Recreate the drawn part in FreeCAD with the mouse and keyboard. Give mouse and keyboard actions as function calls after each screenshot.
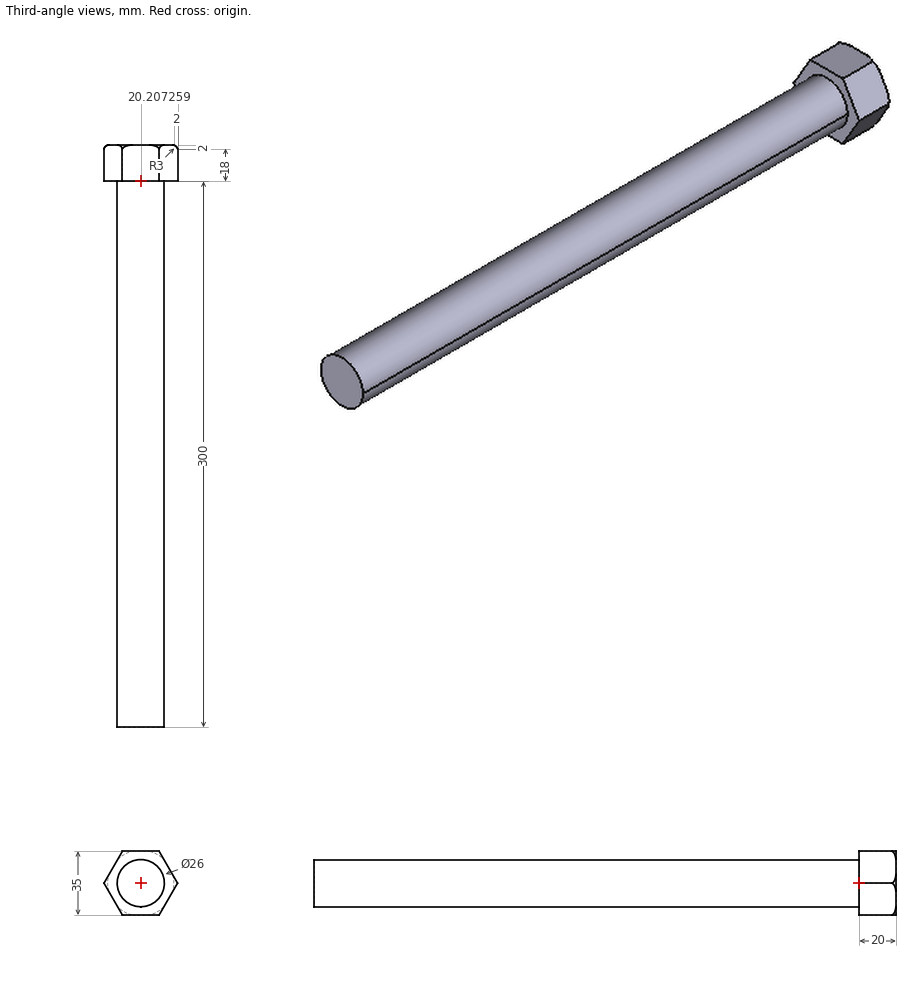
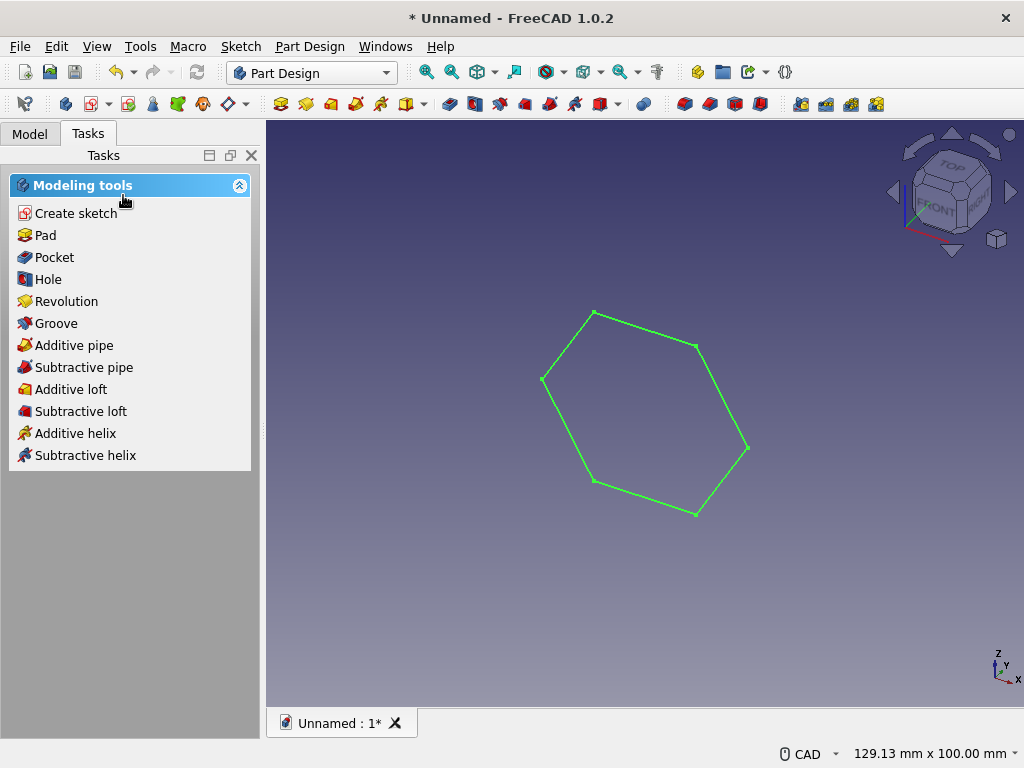
click(281, 104)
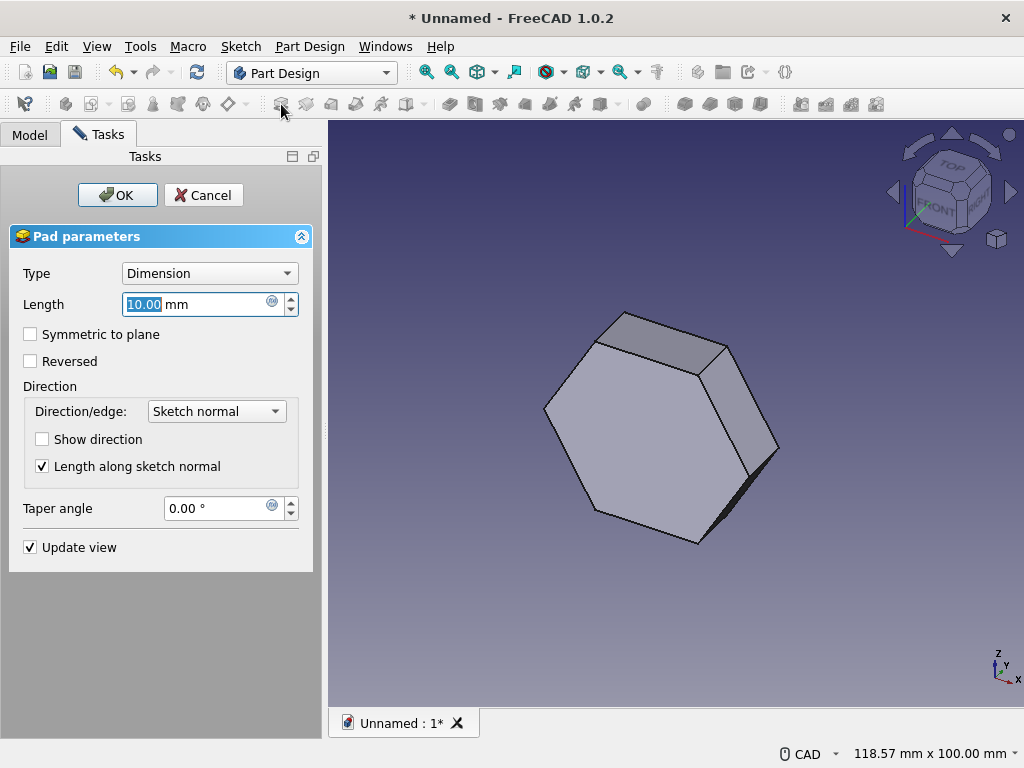
text(20)
key(Tab)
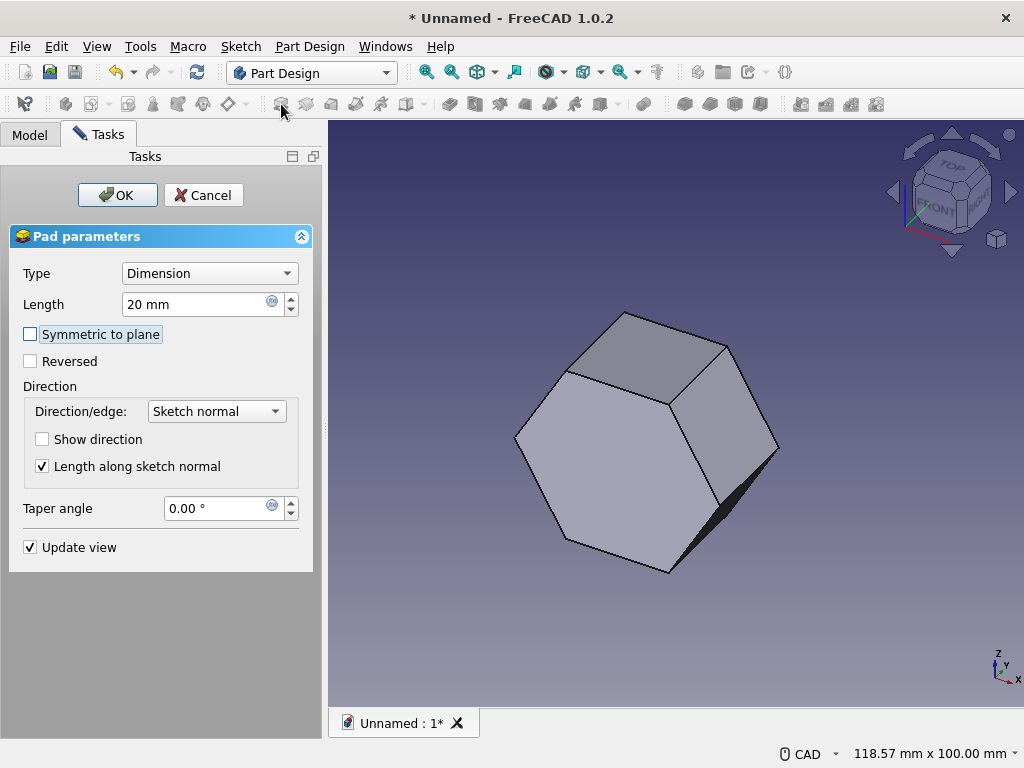
click(31, 361)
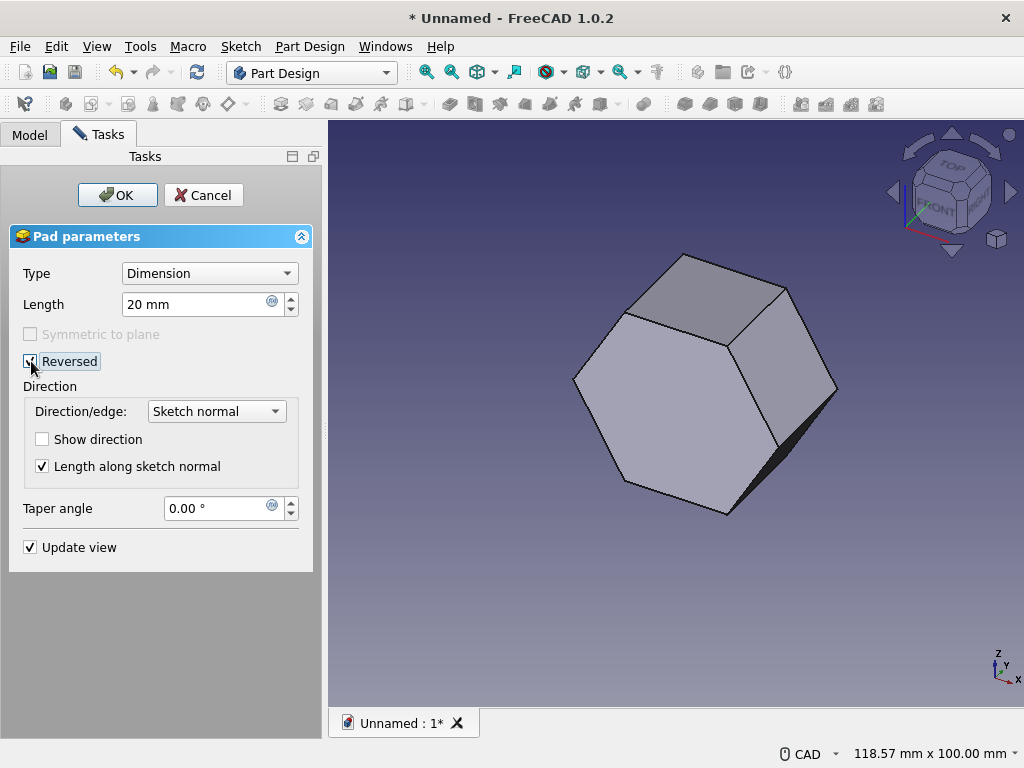
click(118, 195)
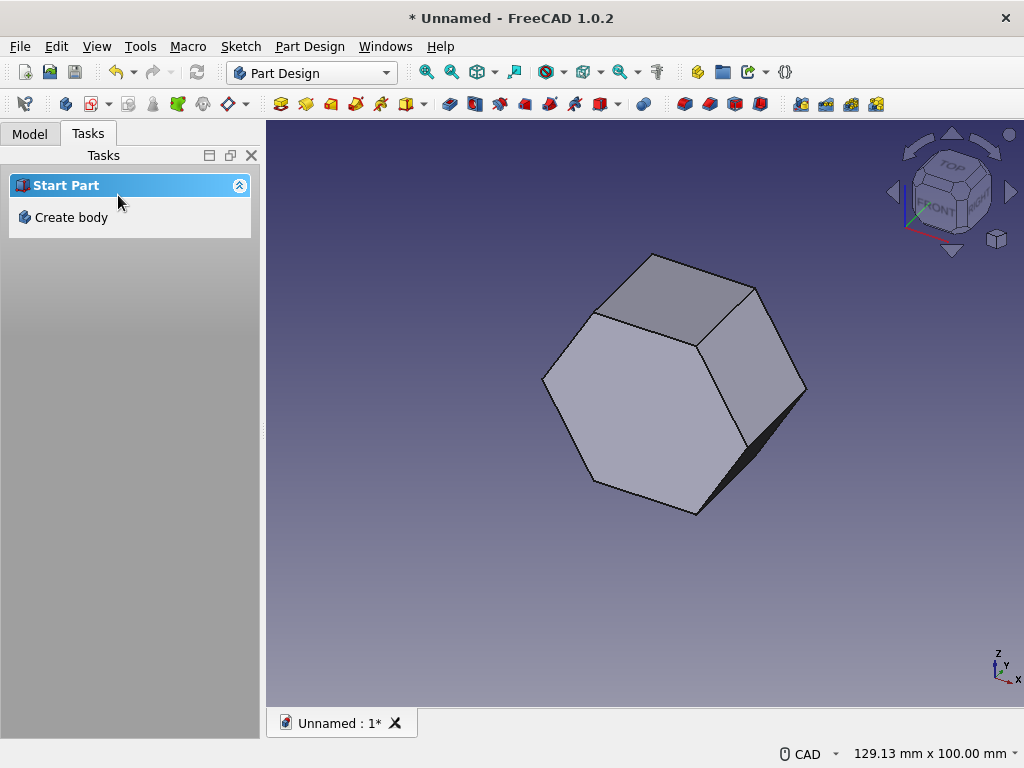
click(90, 104)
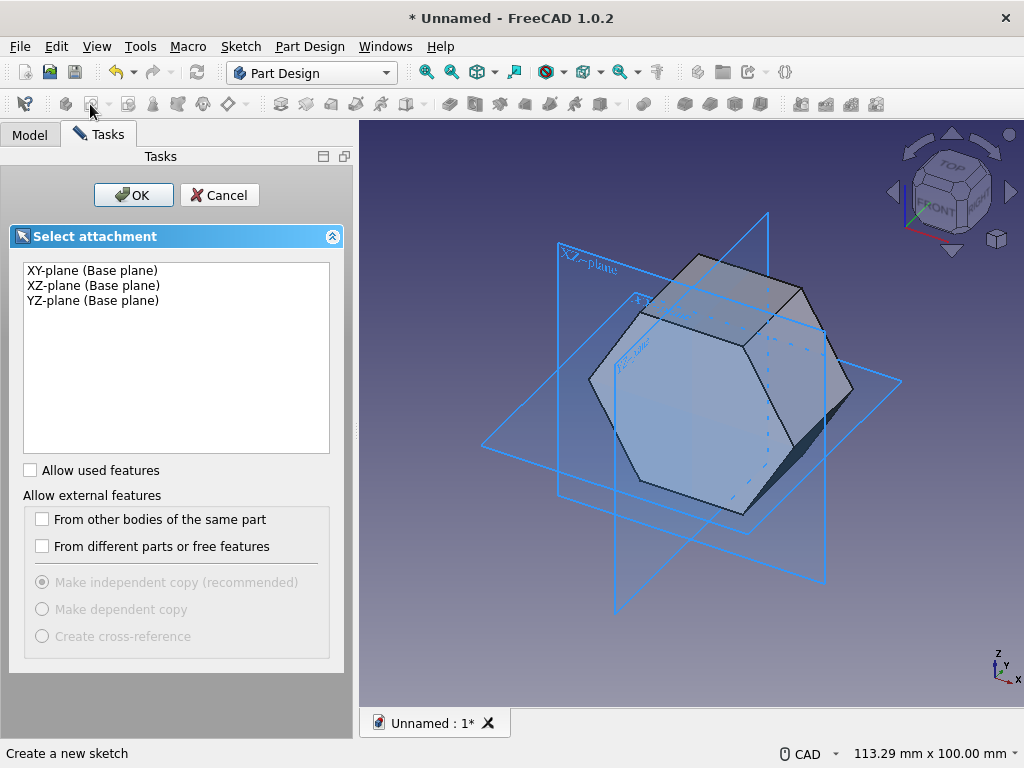
click(84, 286)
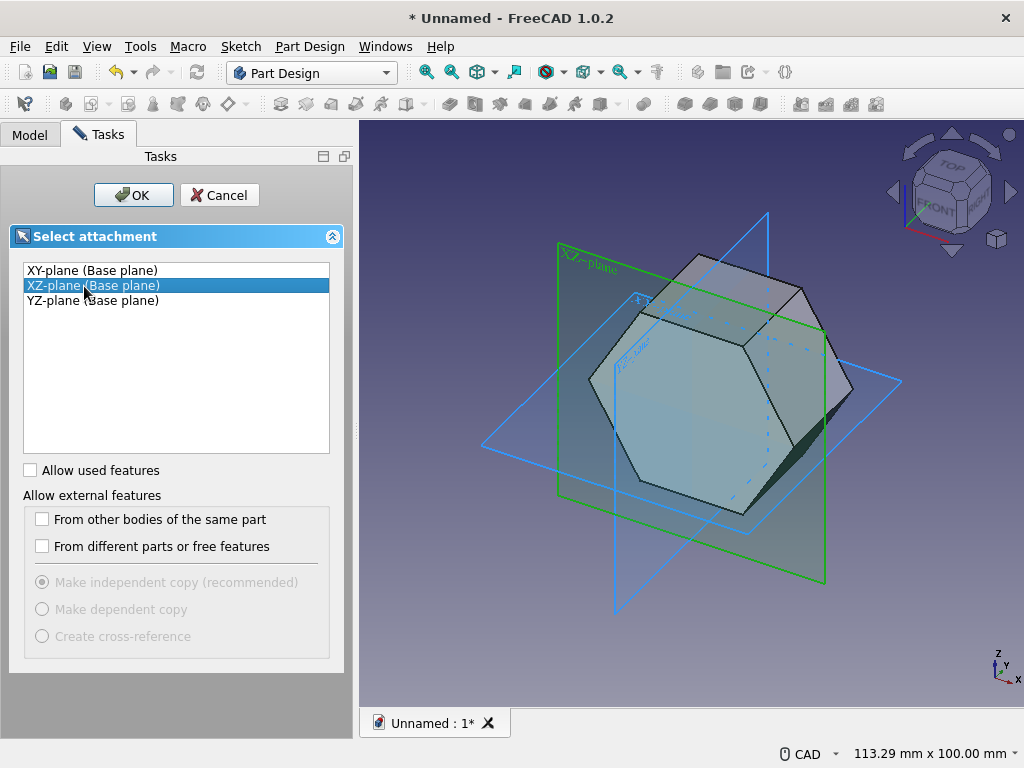
click(134, 195)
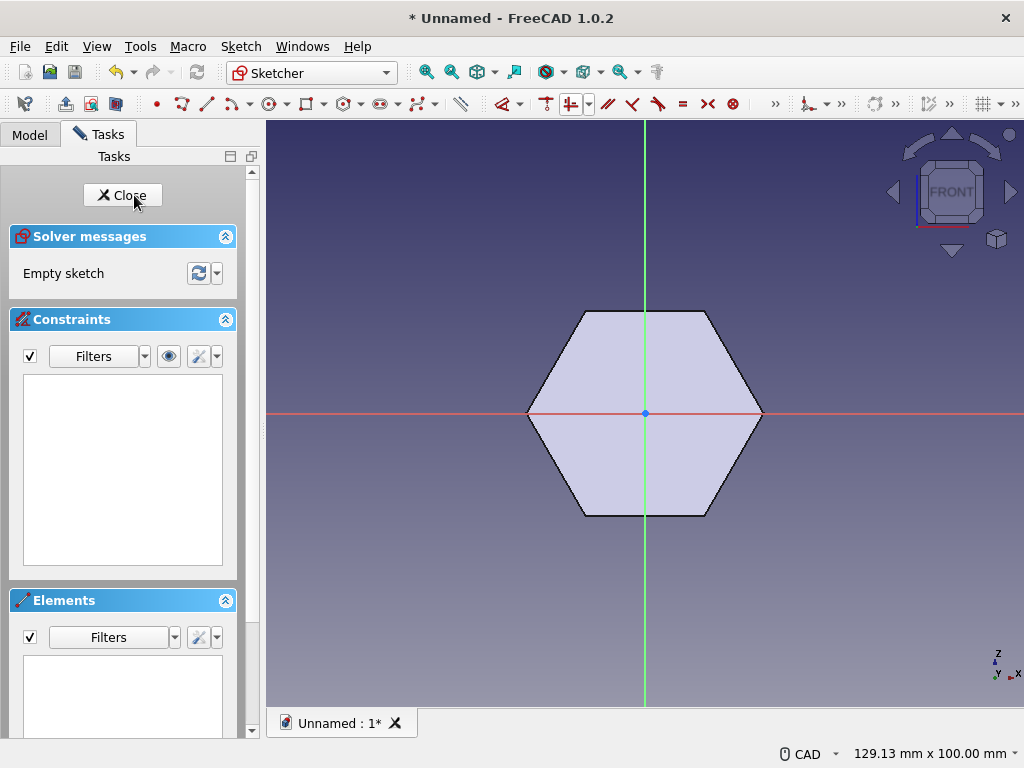
scroll(701, 413, up, 4)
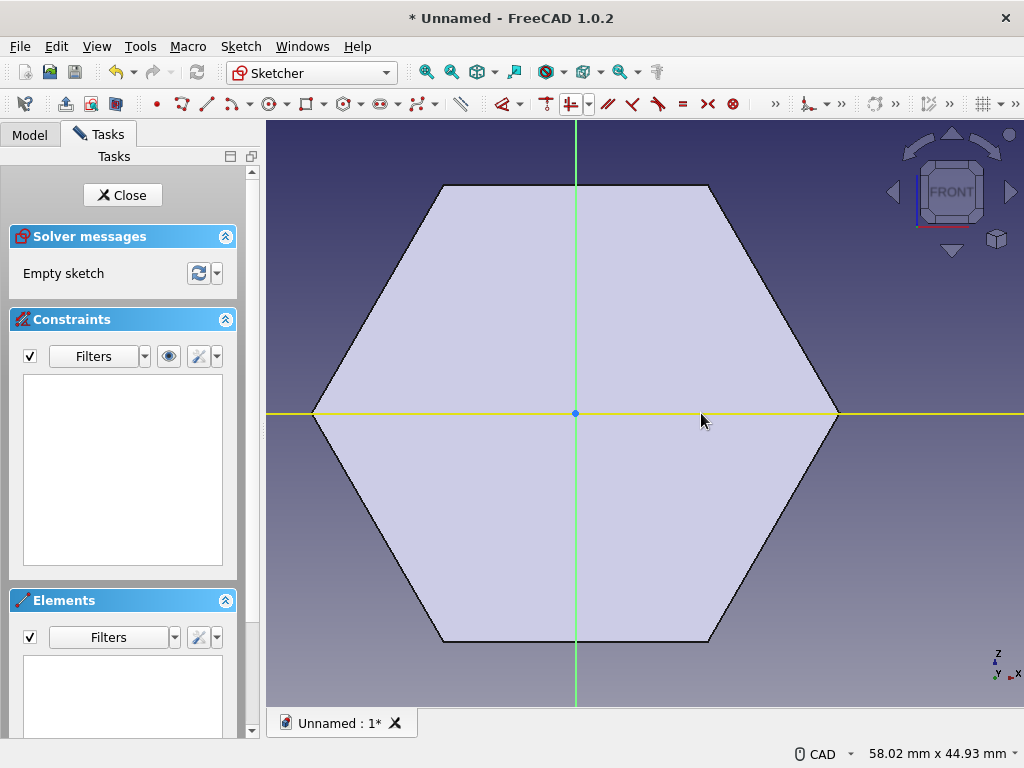
click(268, 104)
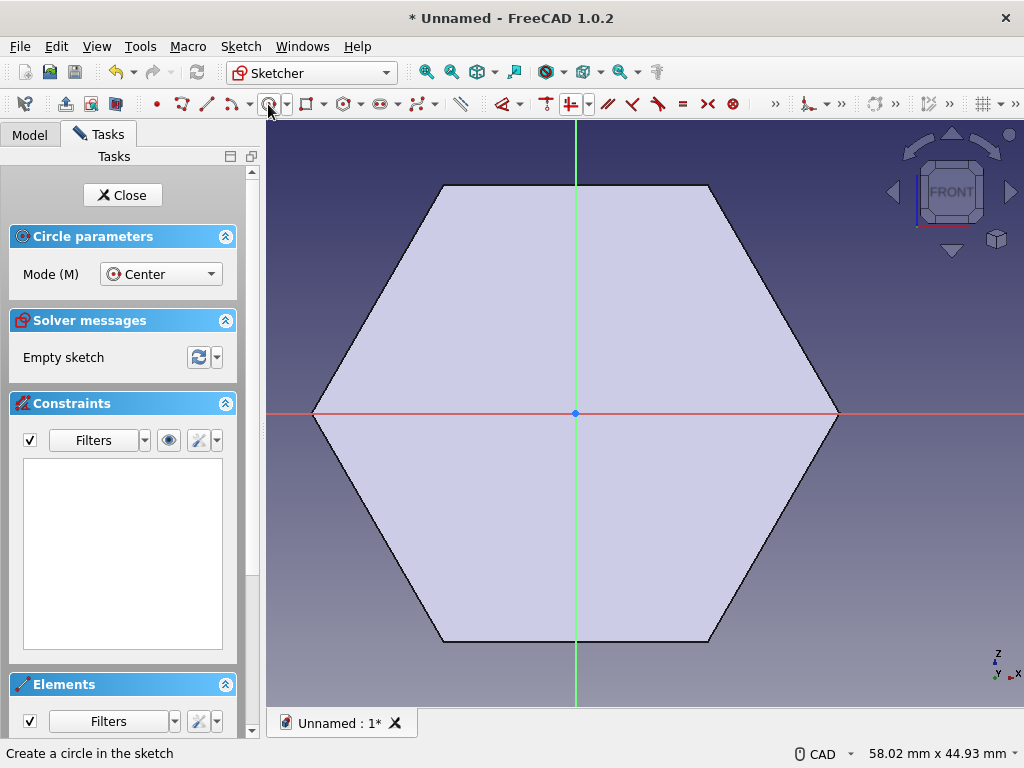
click(576, 414)
move(696, 293)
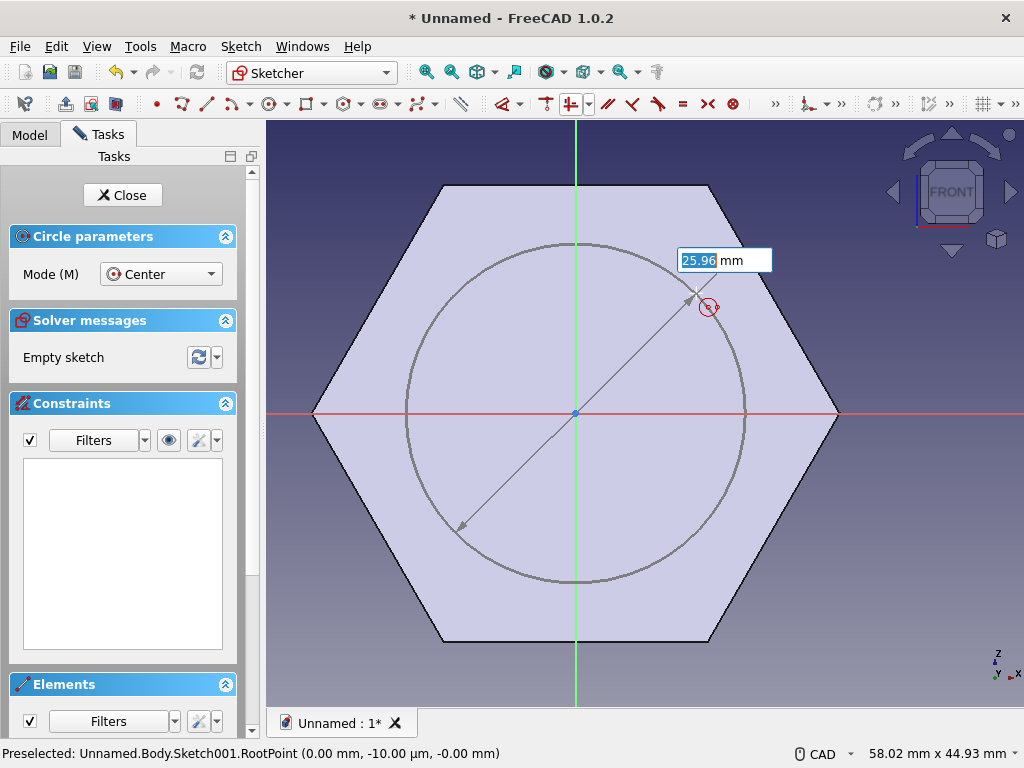
text(26)
key(Return)
key(Escape)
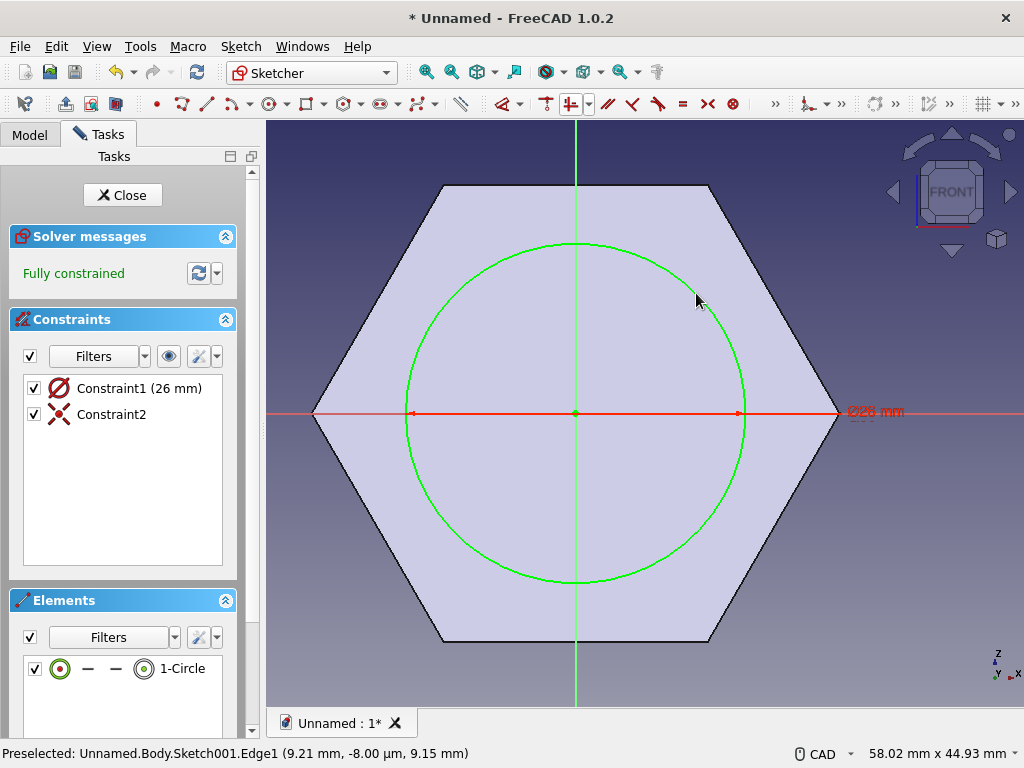
click(123, 195)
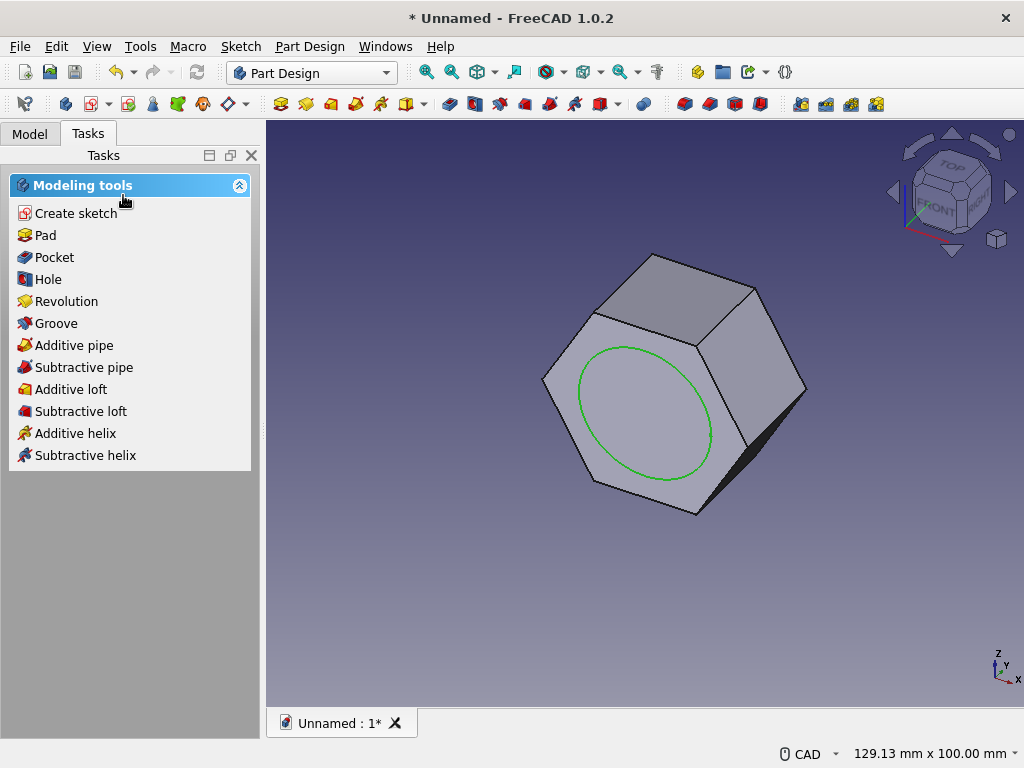
click(281, 104)